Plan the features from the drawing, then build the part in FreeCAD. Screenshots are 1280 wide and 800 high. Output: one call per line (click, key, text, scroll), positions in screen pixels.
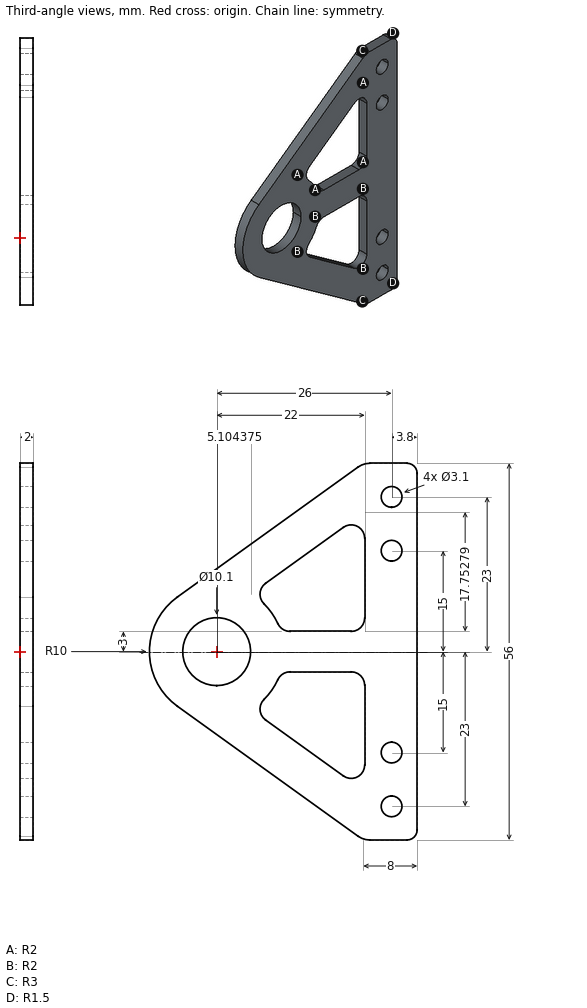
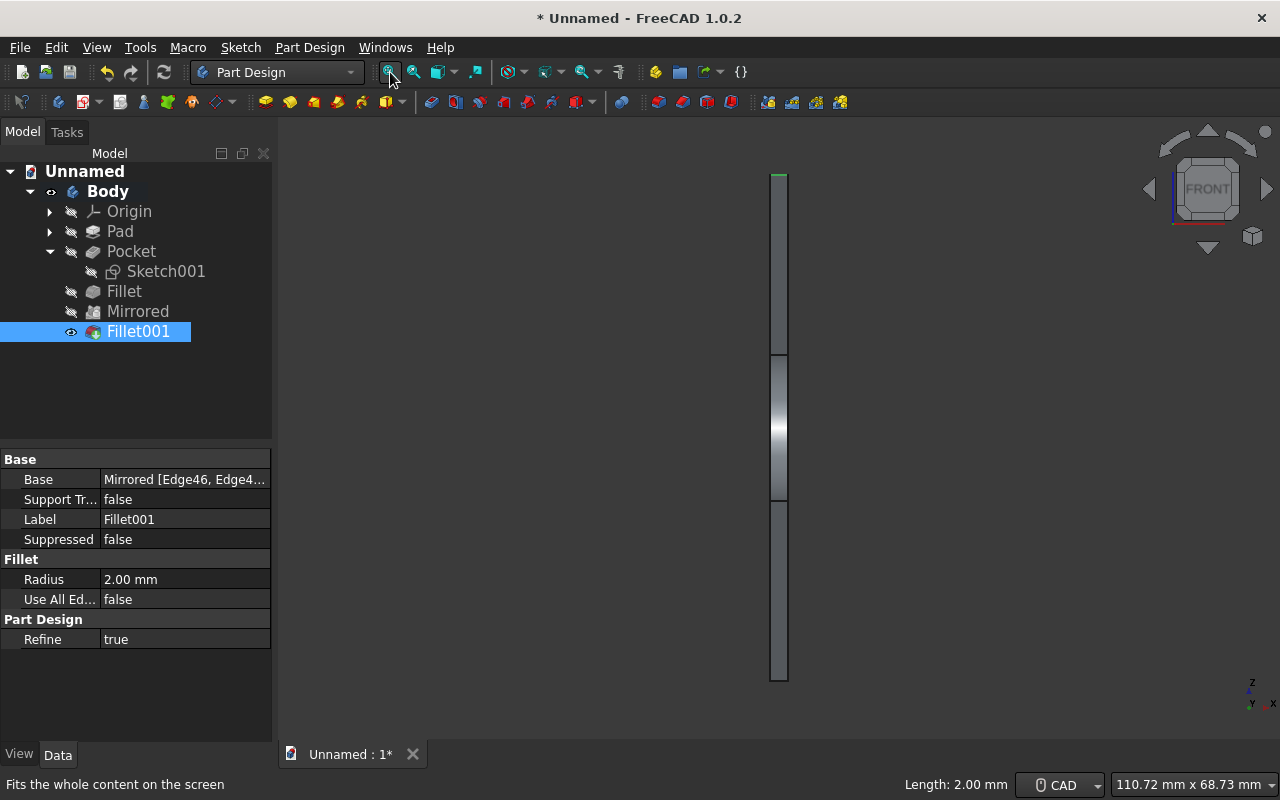
key(3)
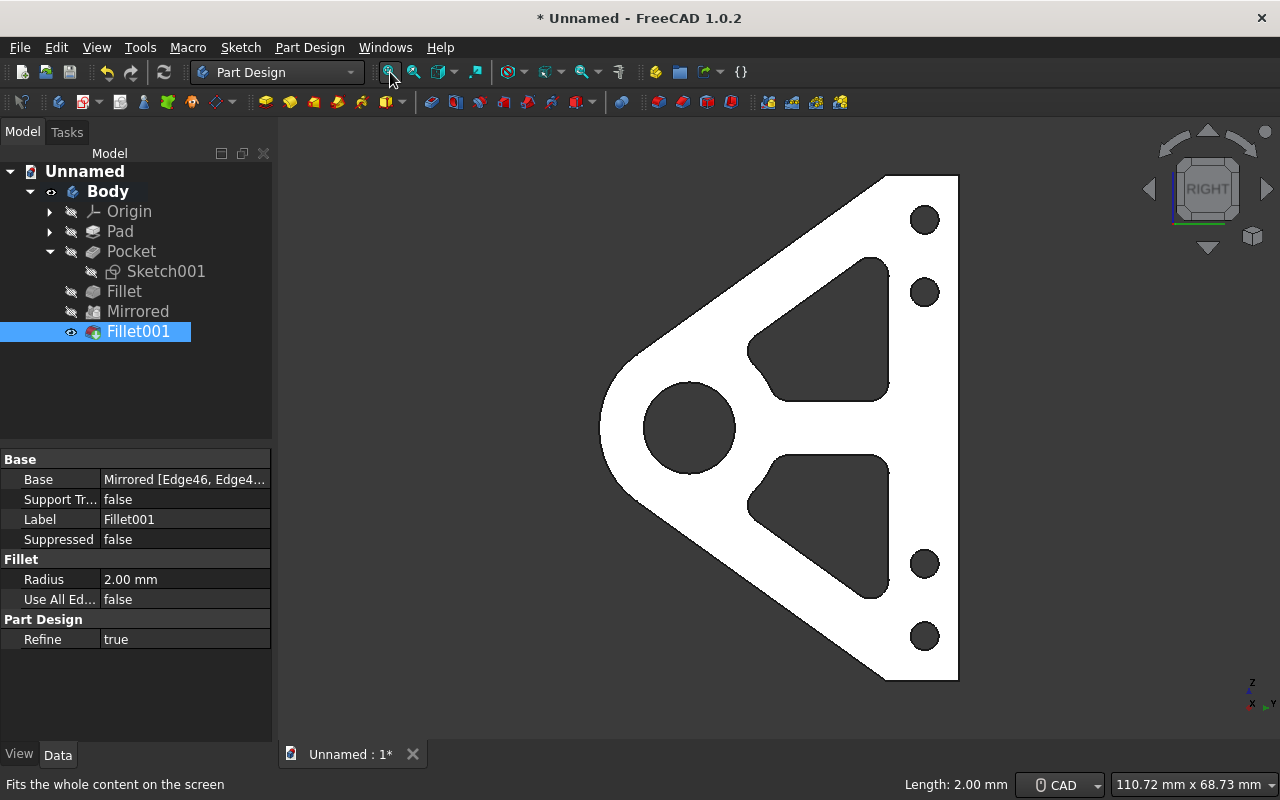
scroll(887, 680, up, 4)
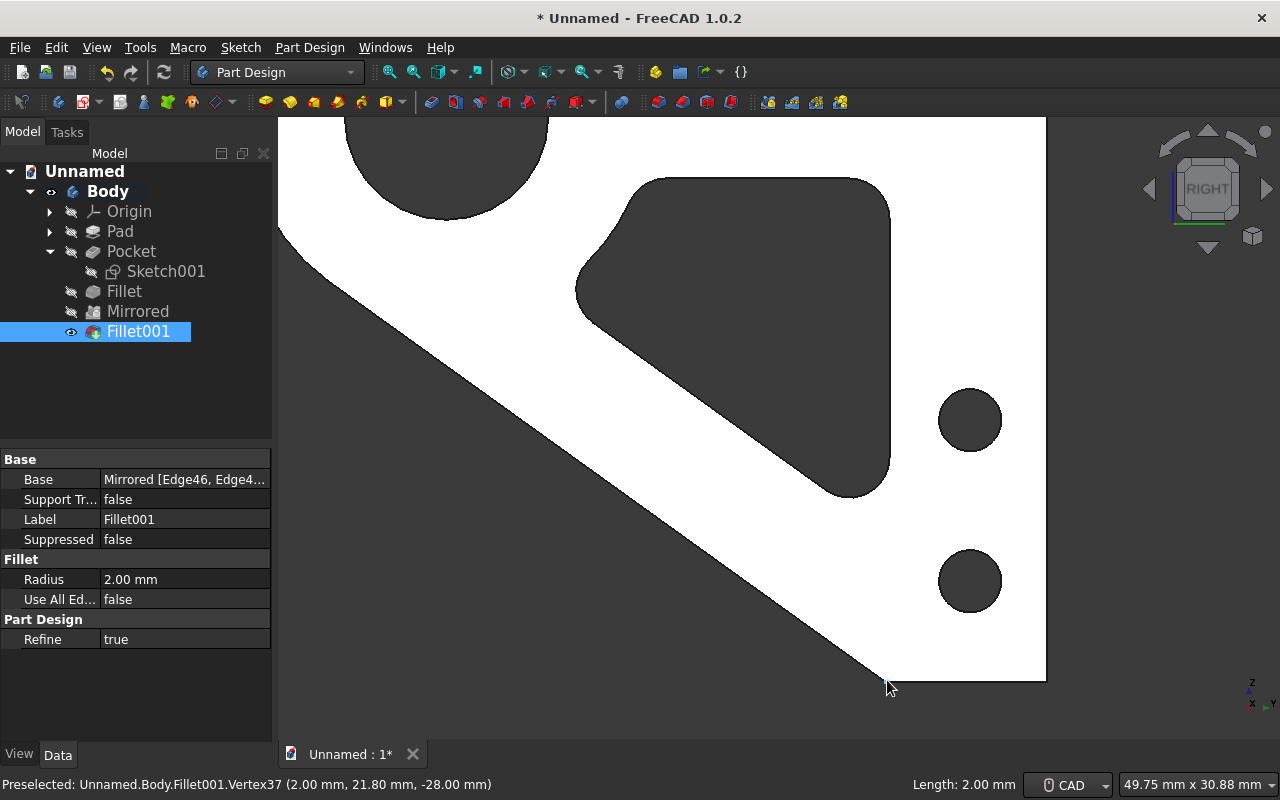
click(390, 72)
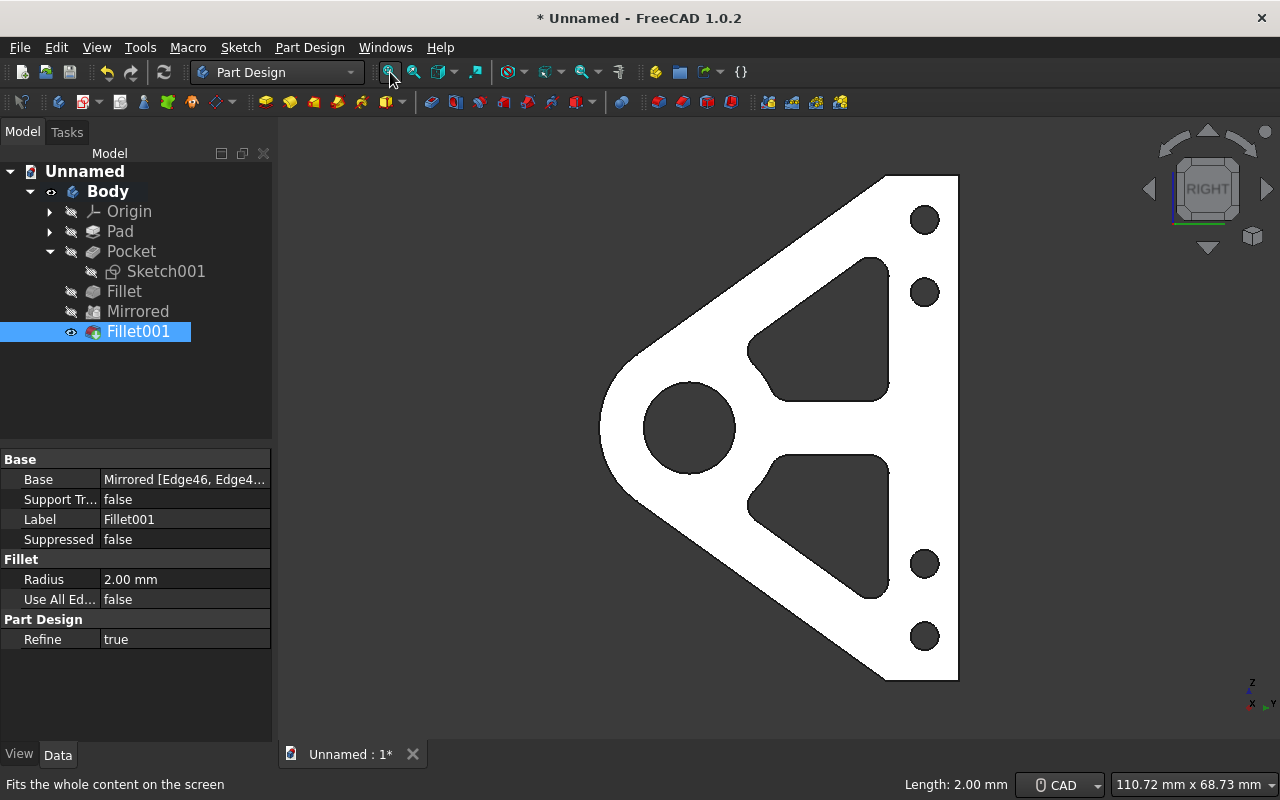
key(5)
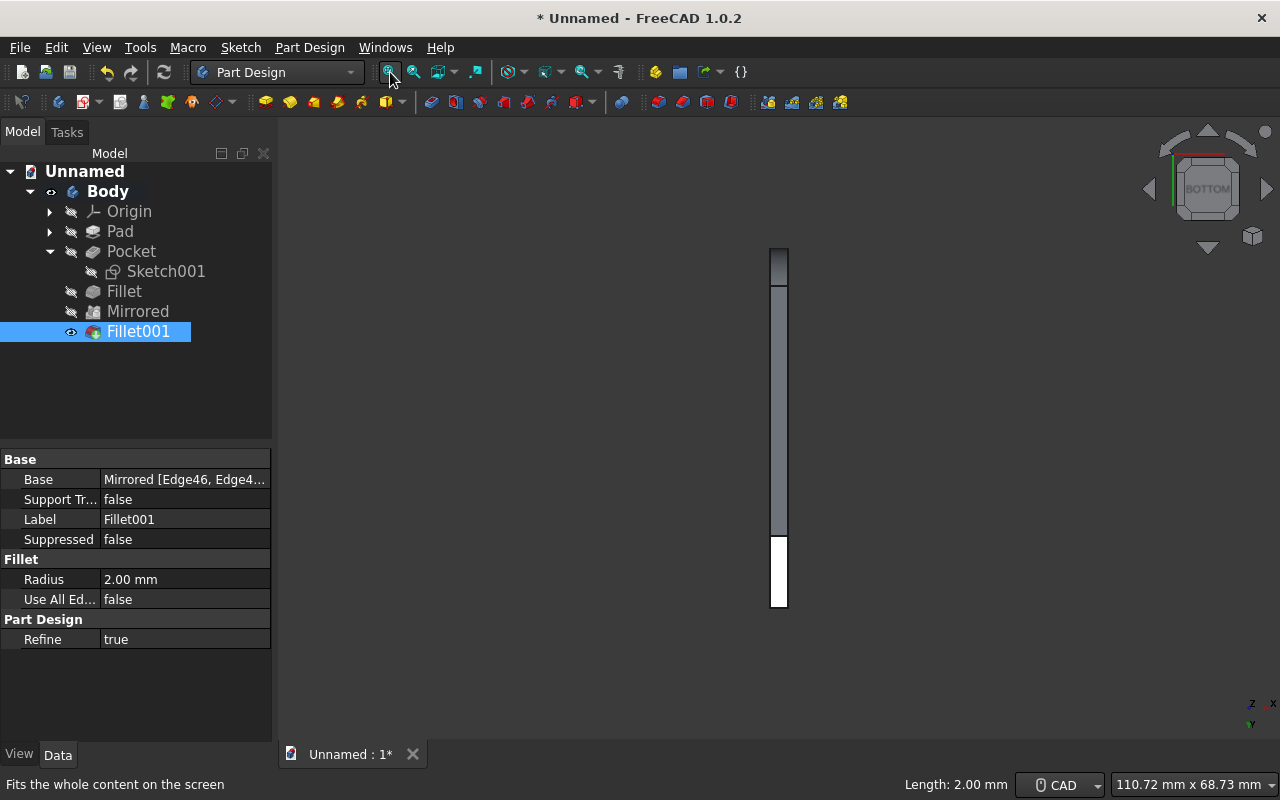
click(779, 535, ctrl)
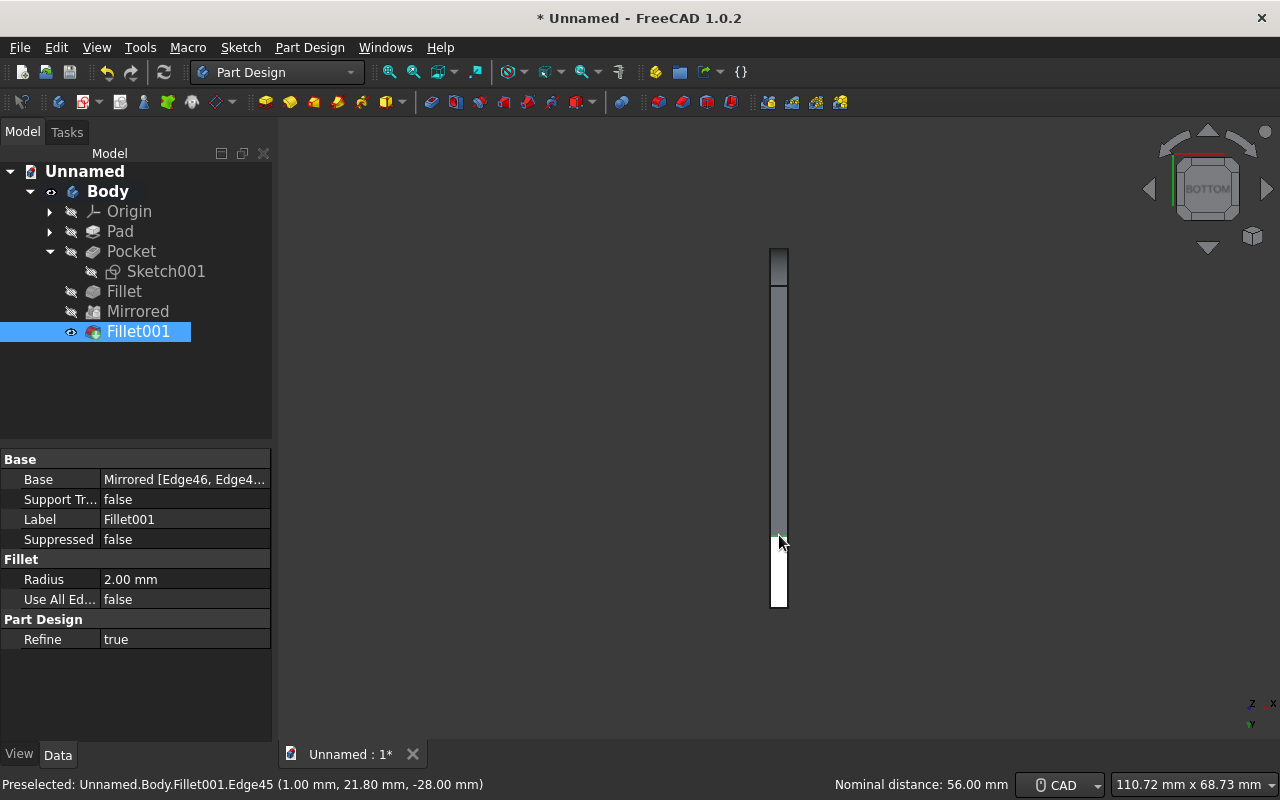
click(660, 102)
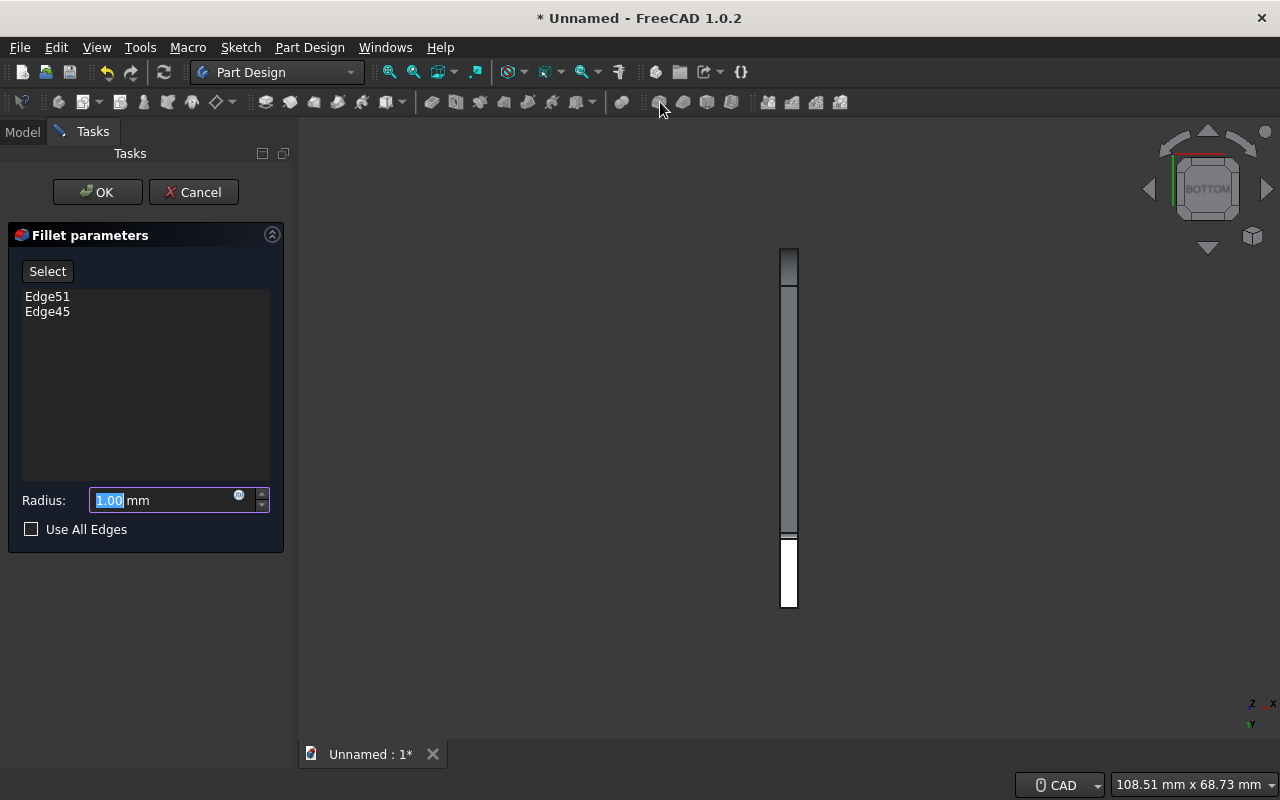
text(3)
key(Tab)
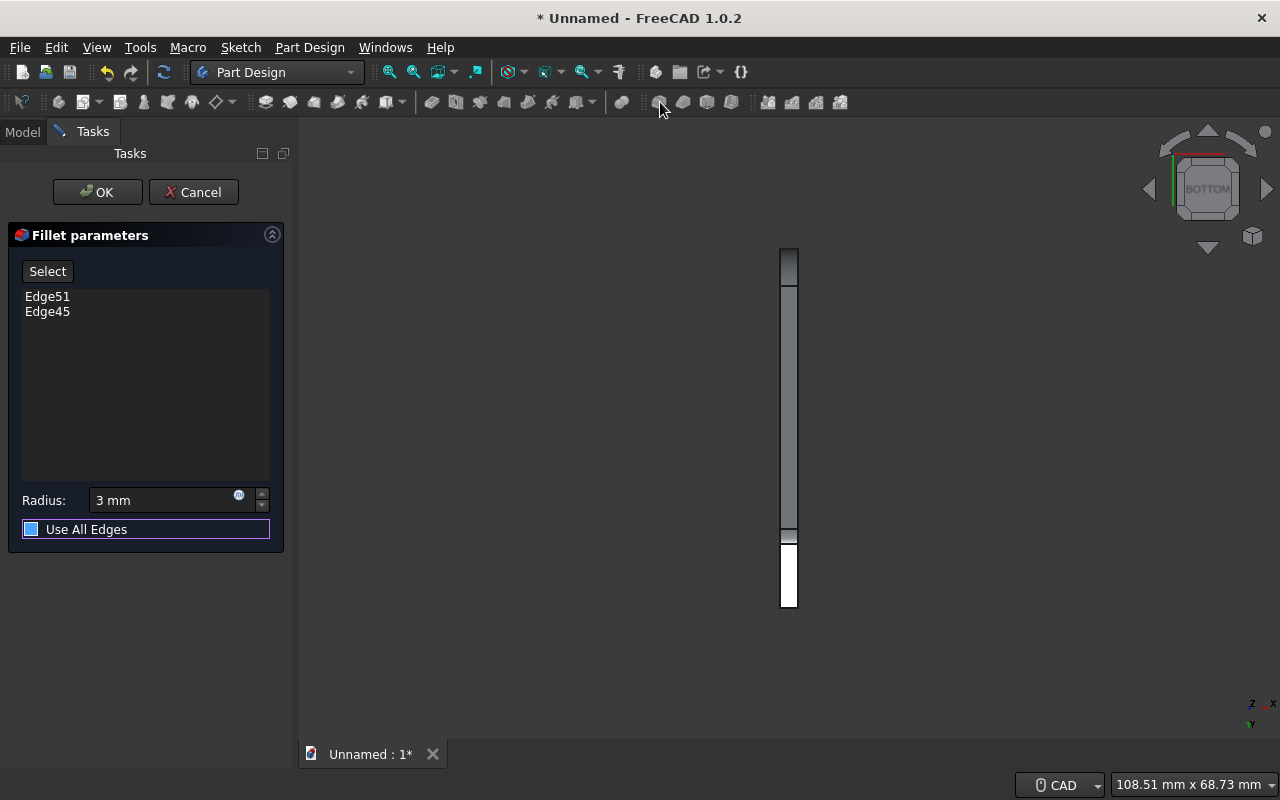
click(98, 192)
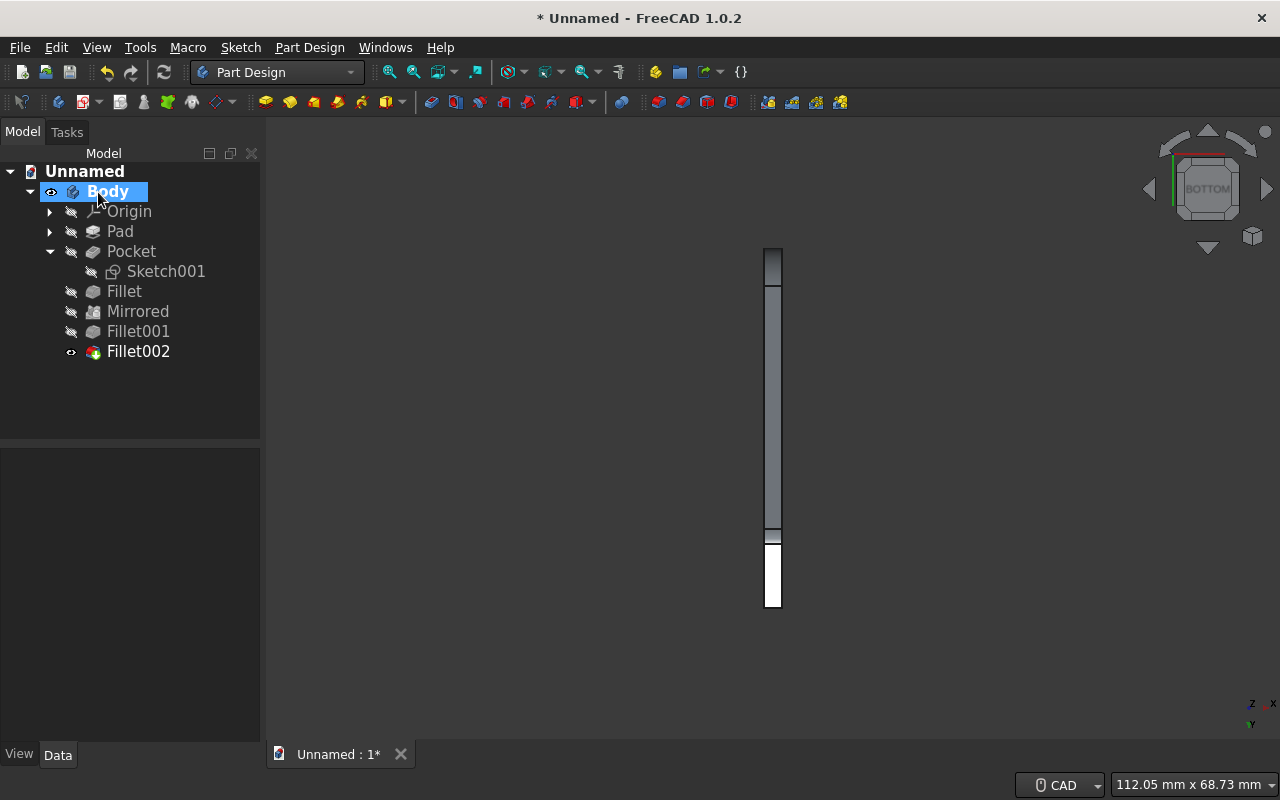
click(773, 607)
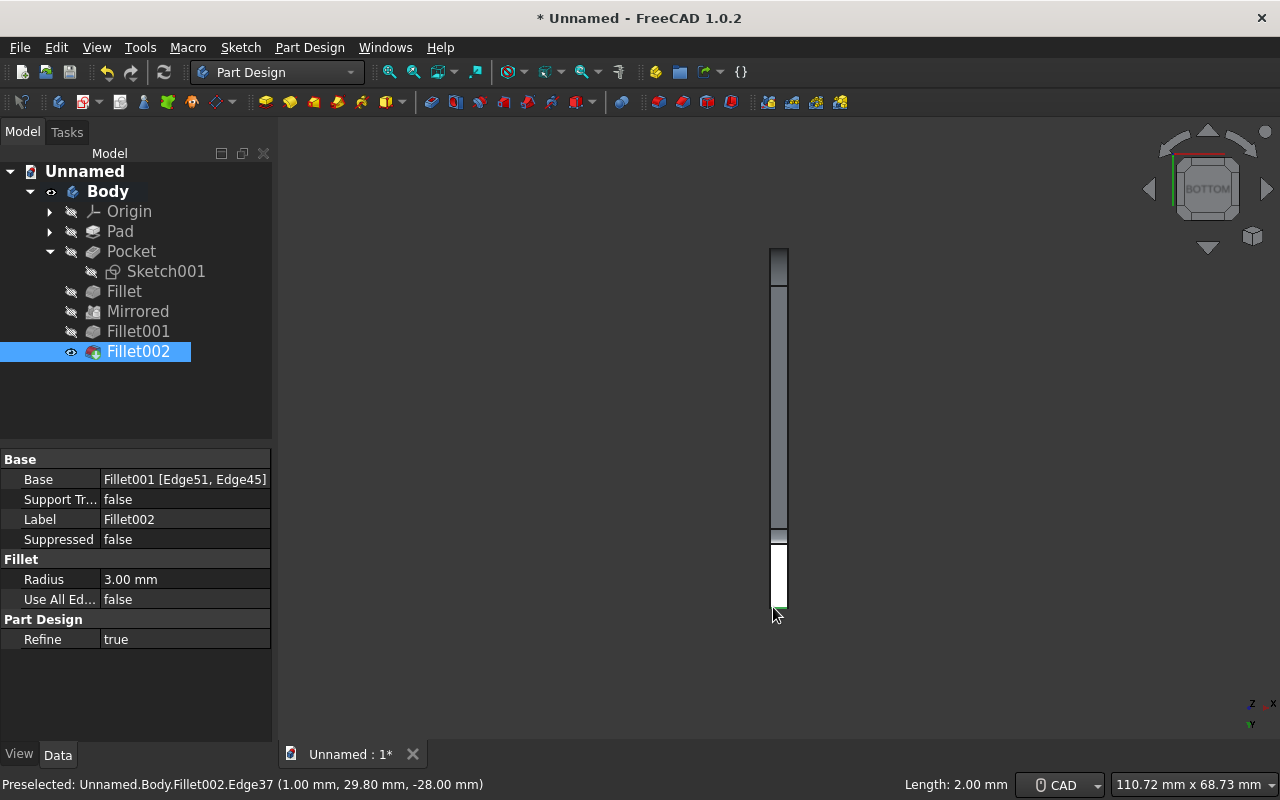
scroll(779, 607, up, 4)